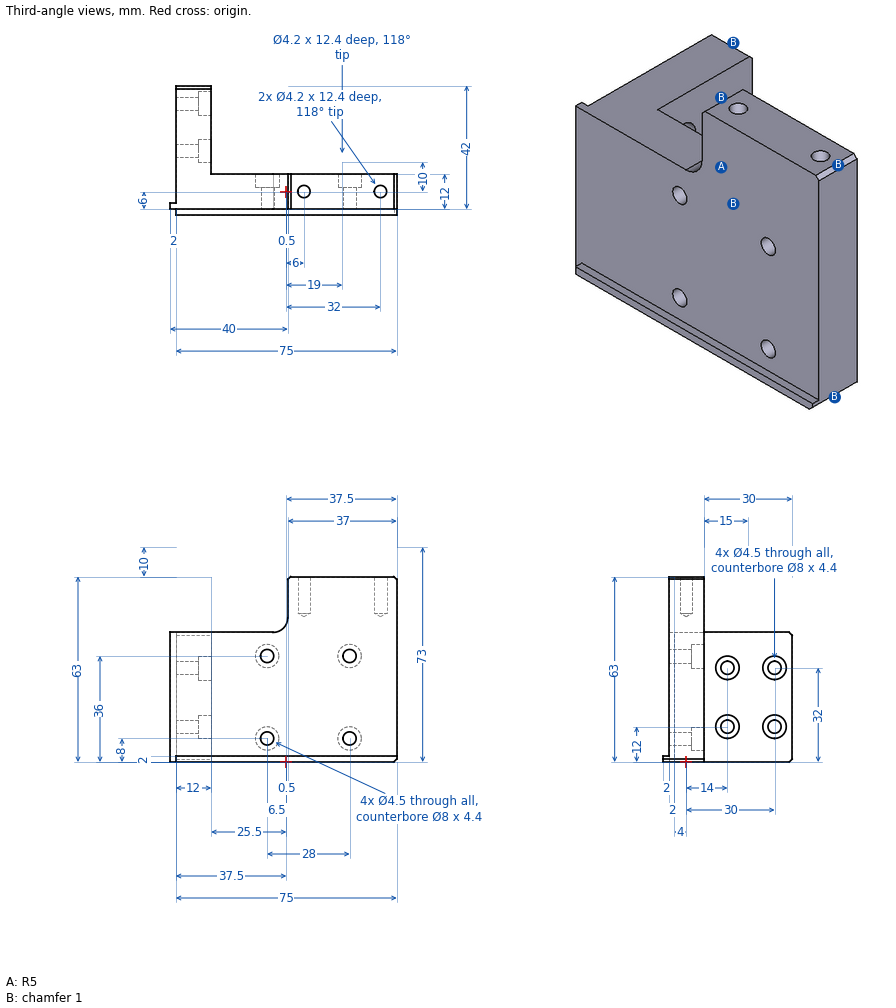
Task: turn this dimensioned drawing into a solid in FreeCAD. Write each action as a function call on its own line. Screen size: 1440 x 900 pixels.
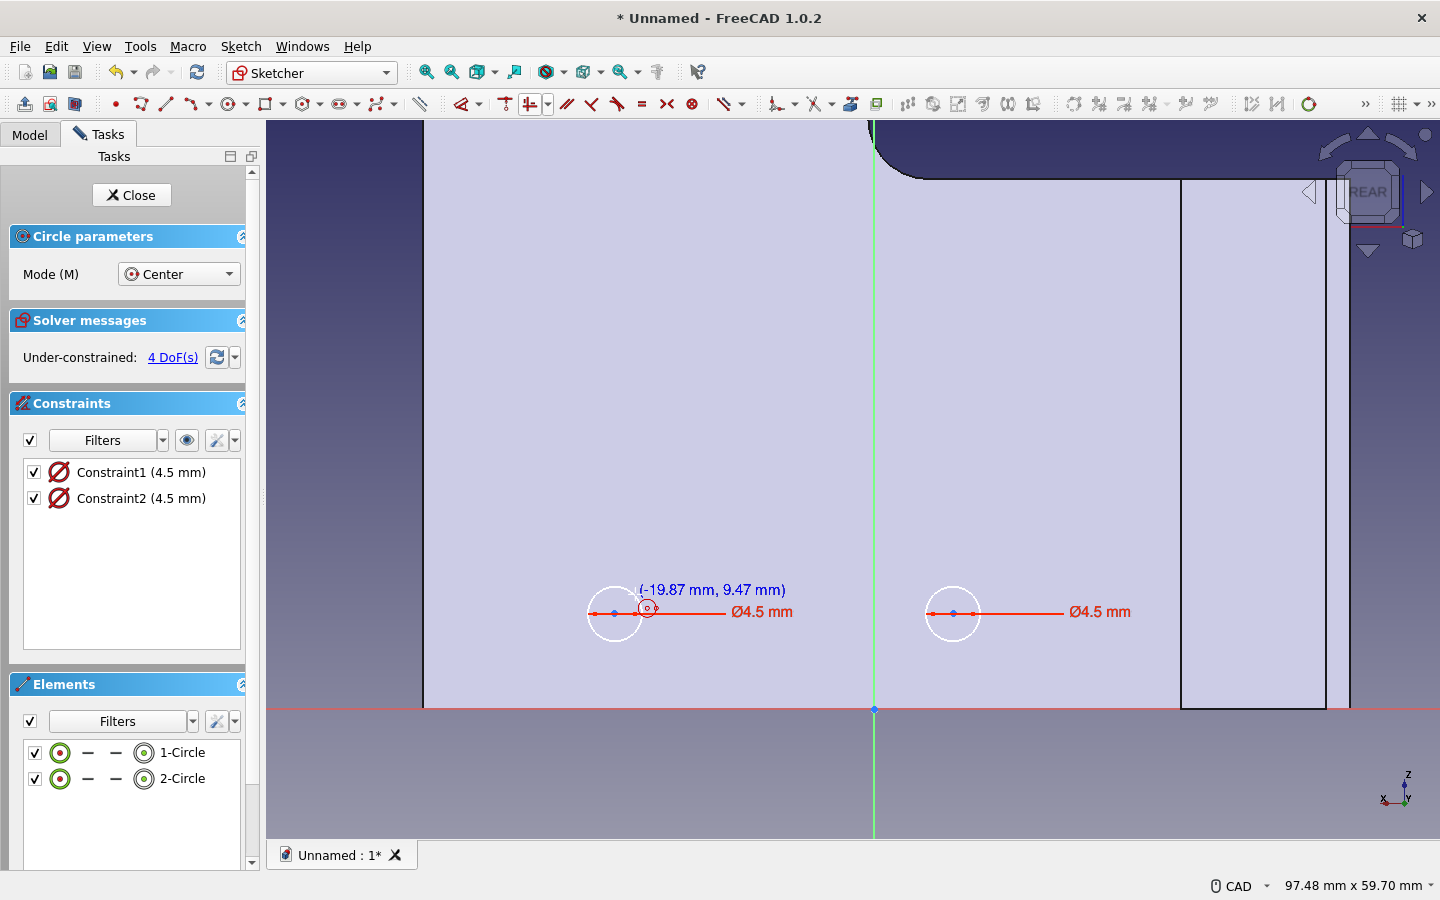
click(953, 275)
move(972, 256)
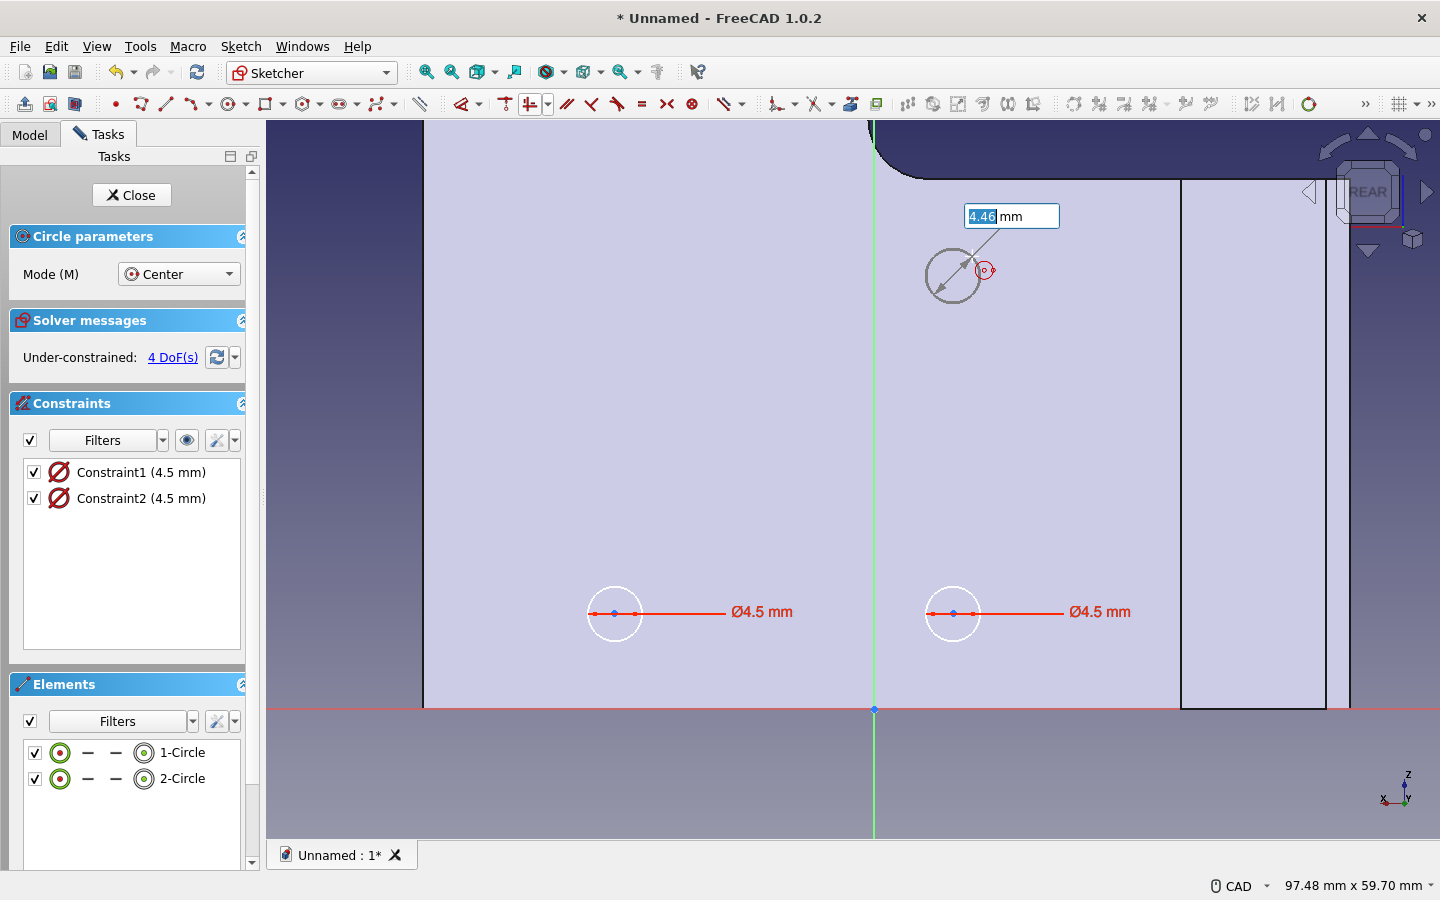
text(4.5)
key(Return)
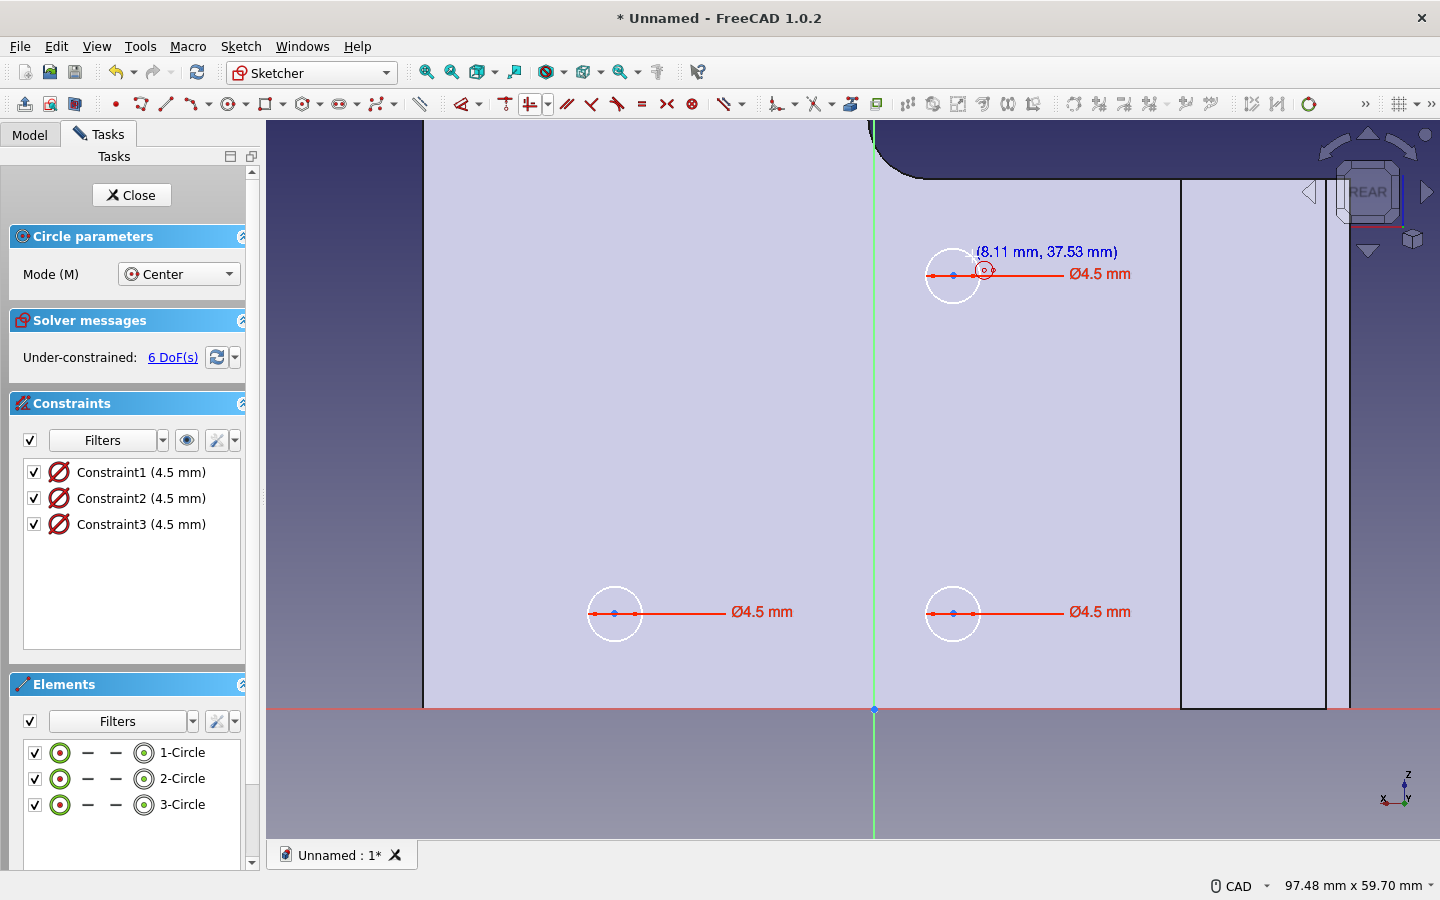
click(615, 275)
move(635, 256)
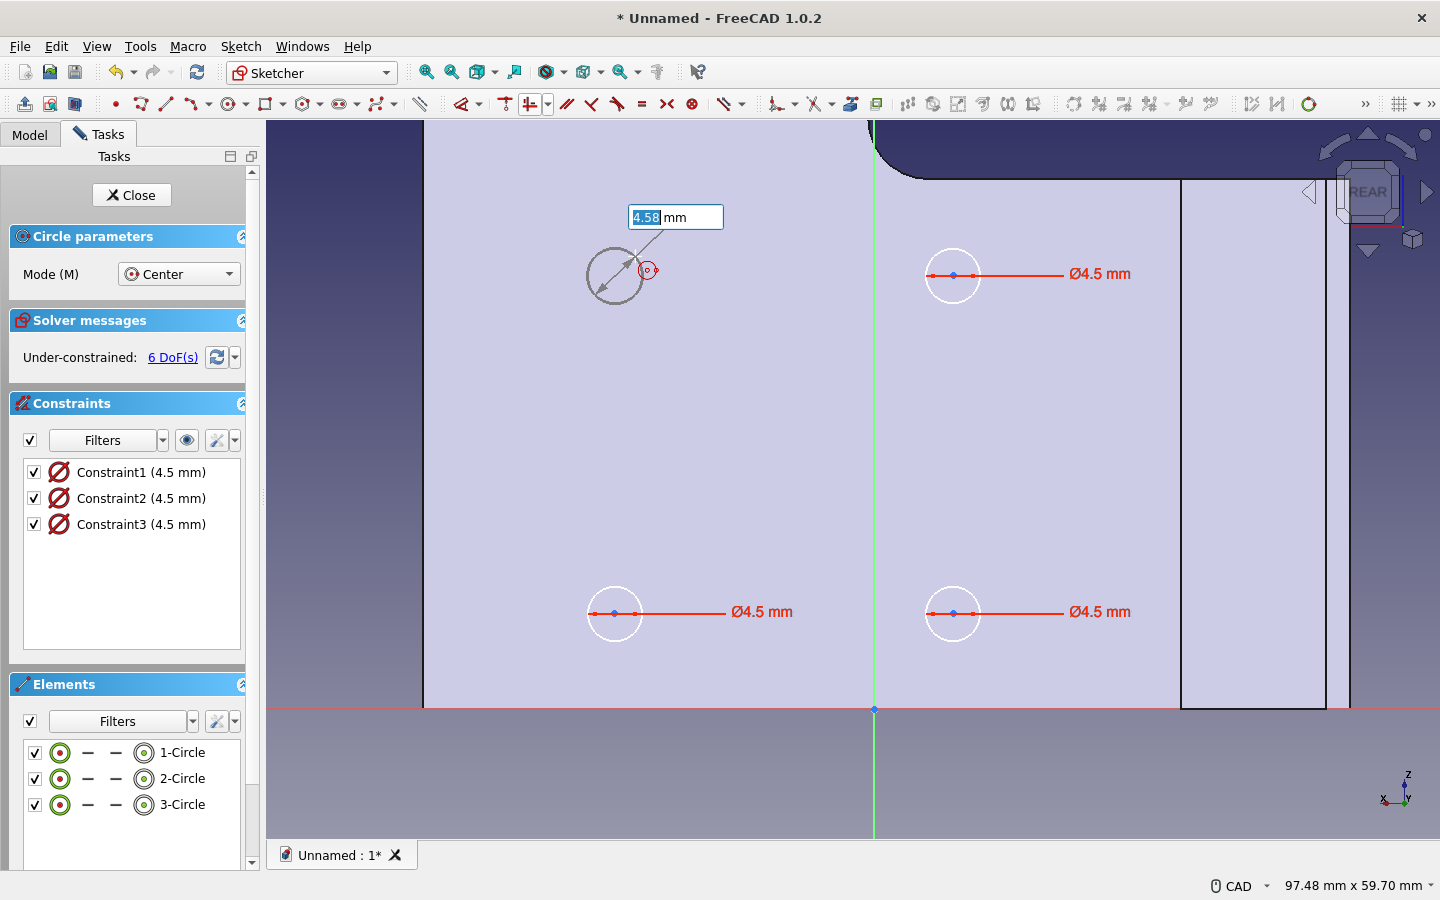
text(4.5)
key(Return)
key(Escape)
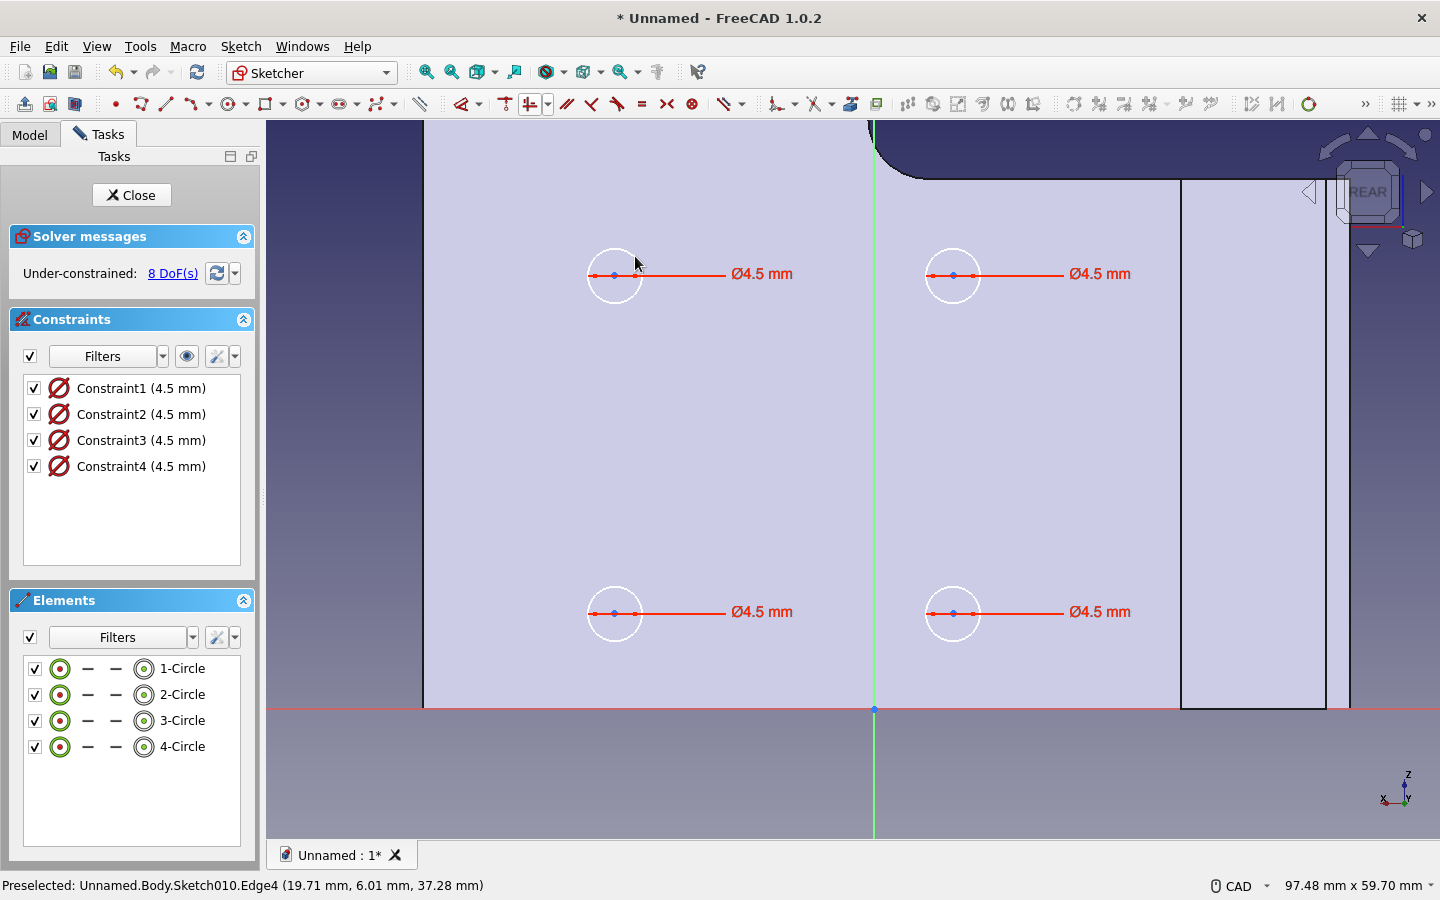
click(953, 614)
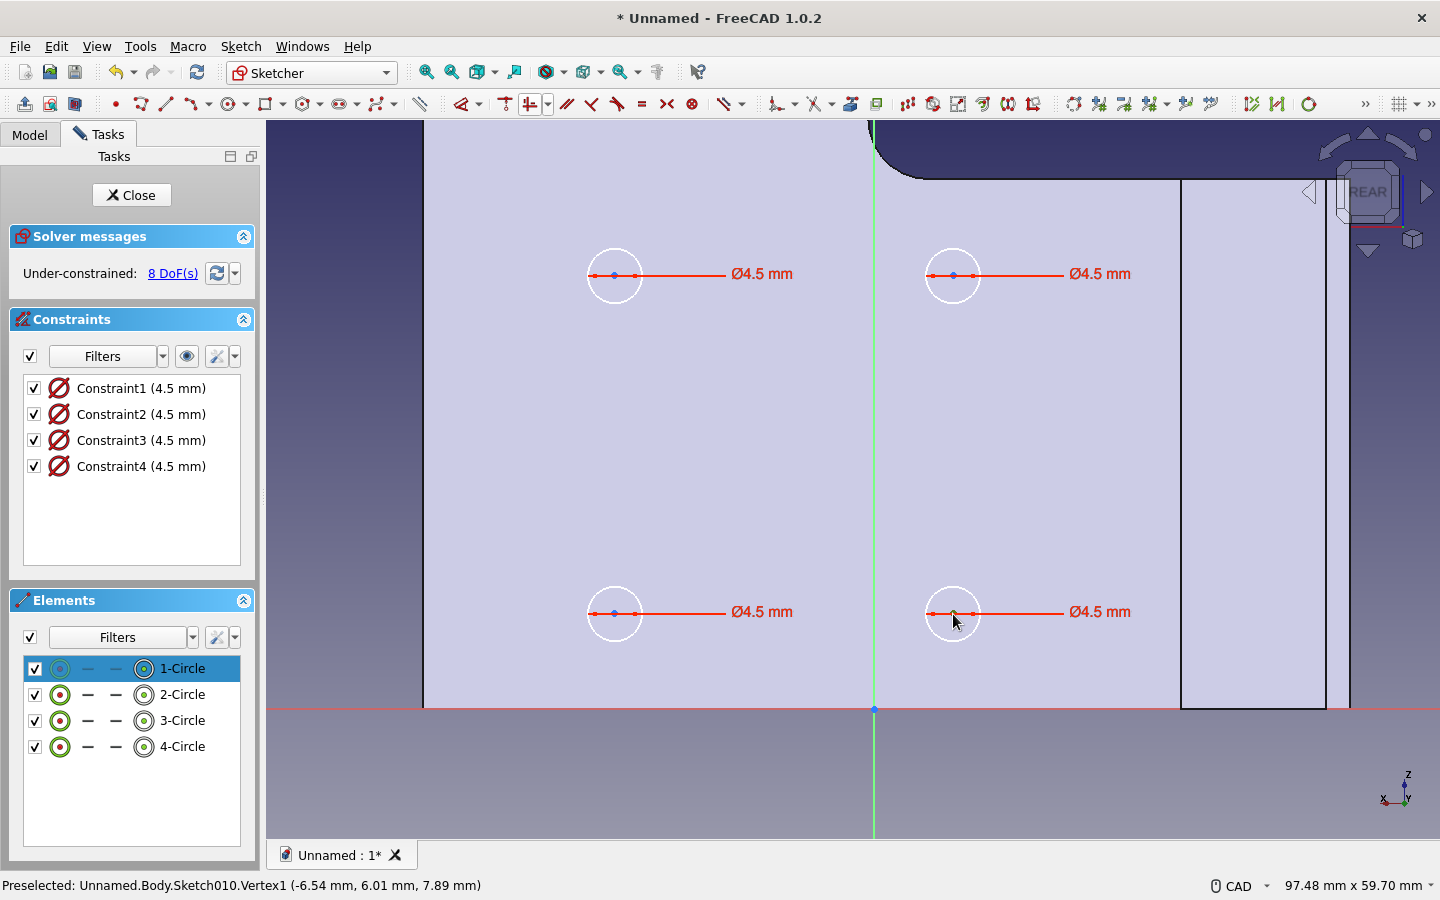
click(615, 614)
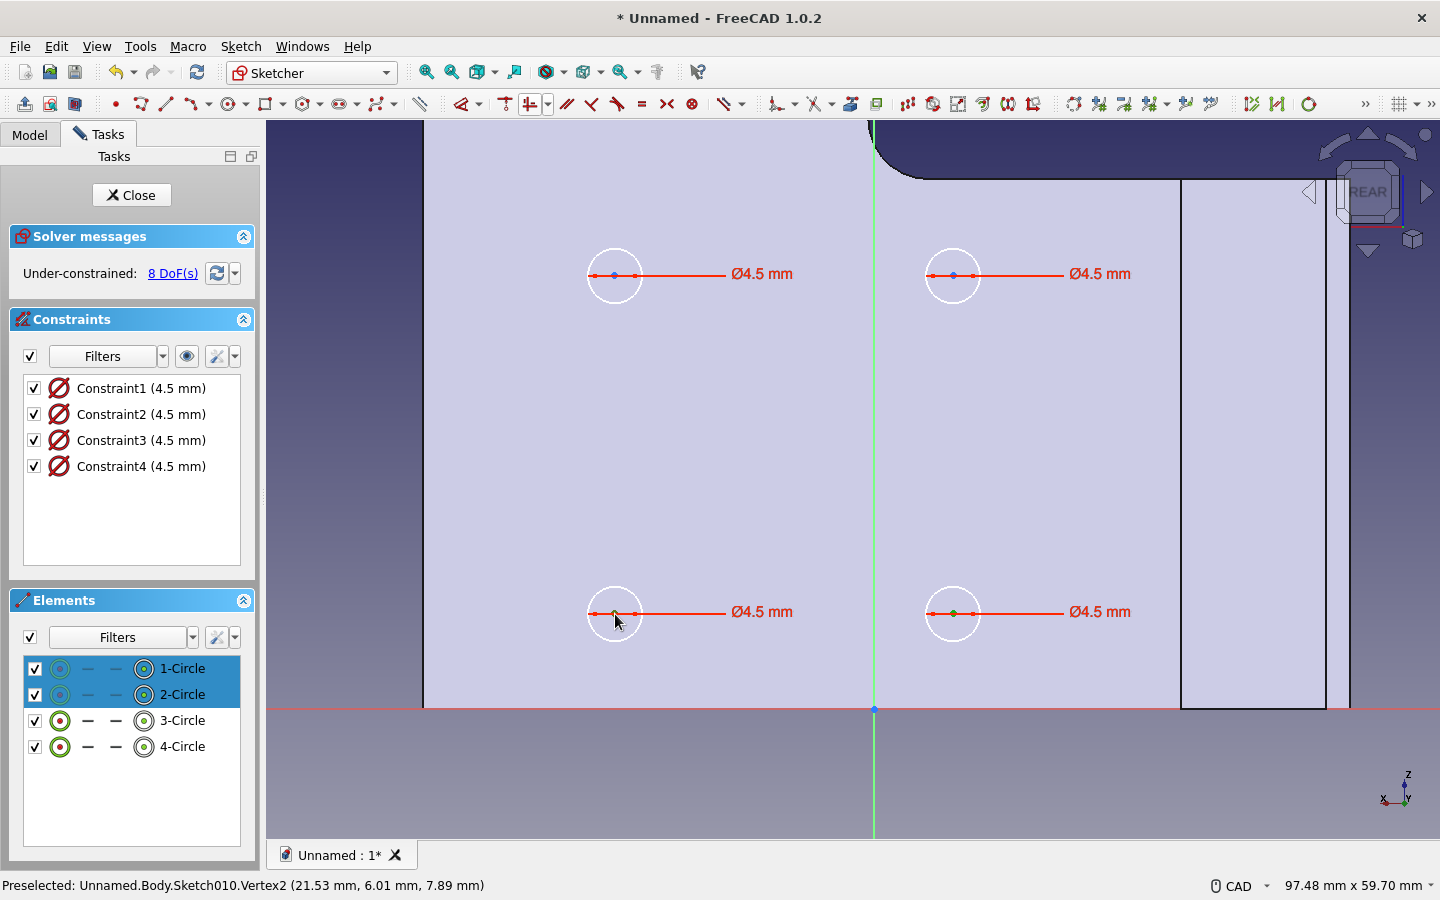
click(548, 104)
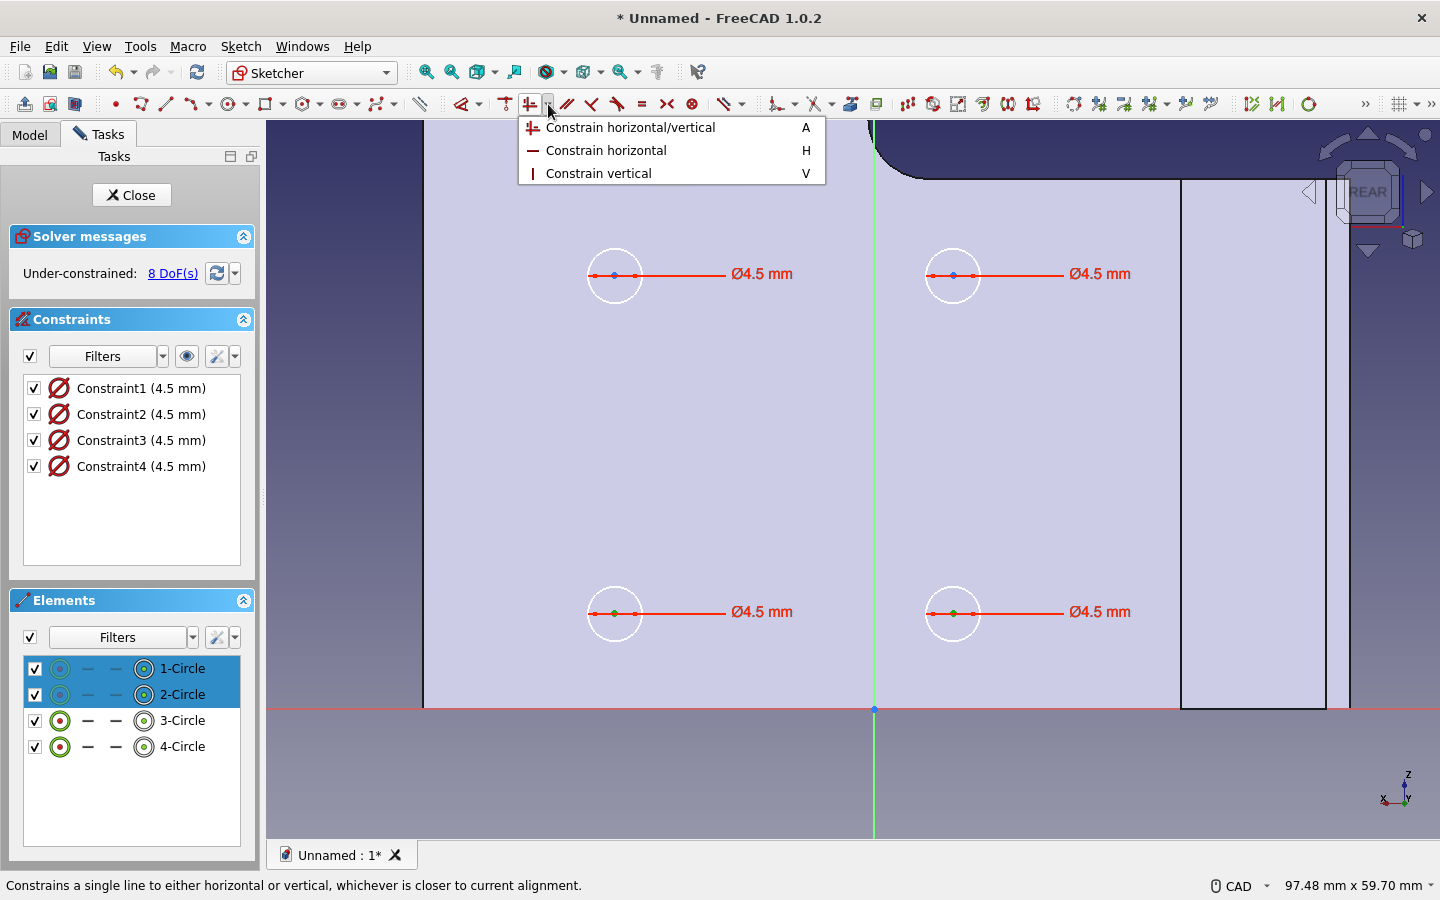
click(672, 150)